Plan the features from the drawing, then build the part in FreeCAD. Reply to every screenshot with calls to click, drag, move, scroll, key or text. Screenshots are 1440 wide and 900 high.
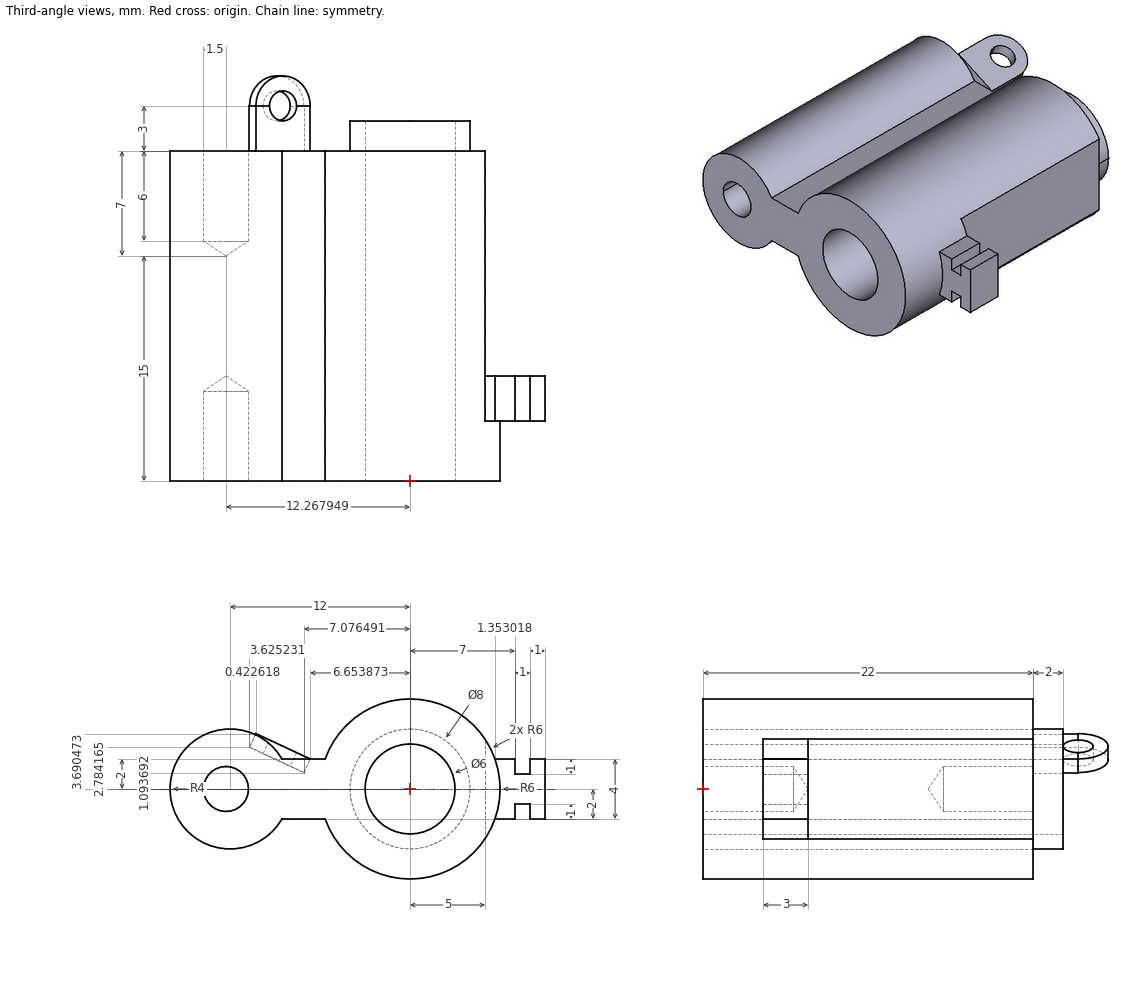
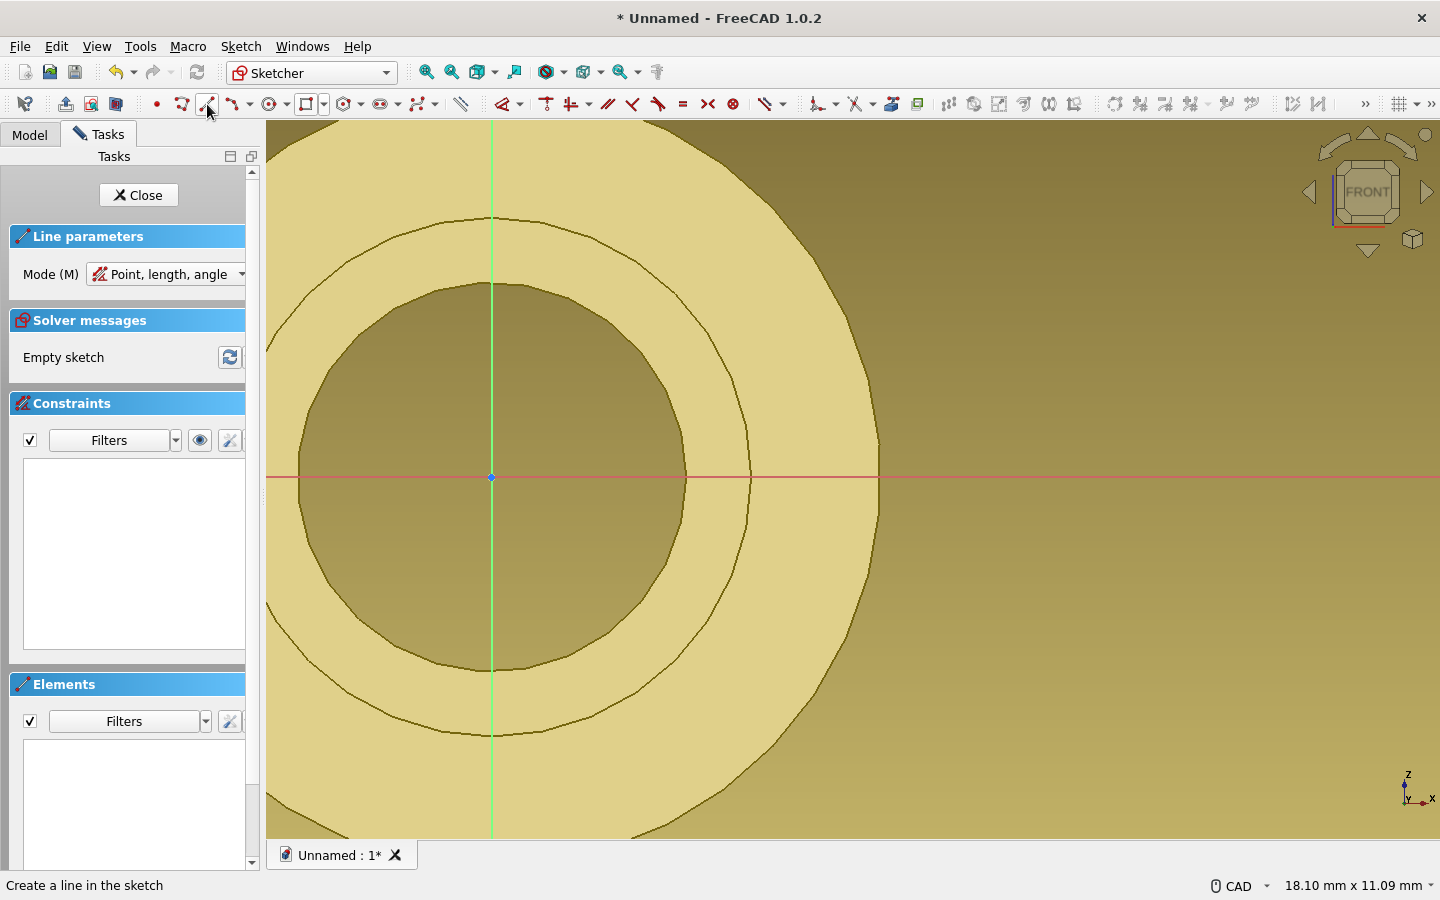
click(816, 692)
click(816, 262)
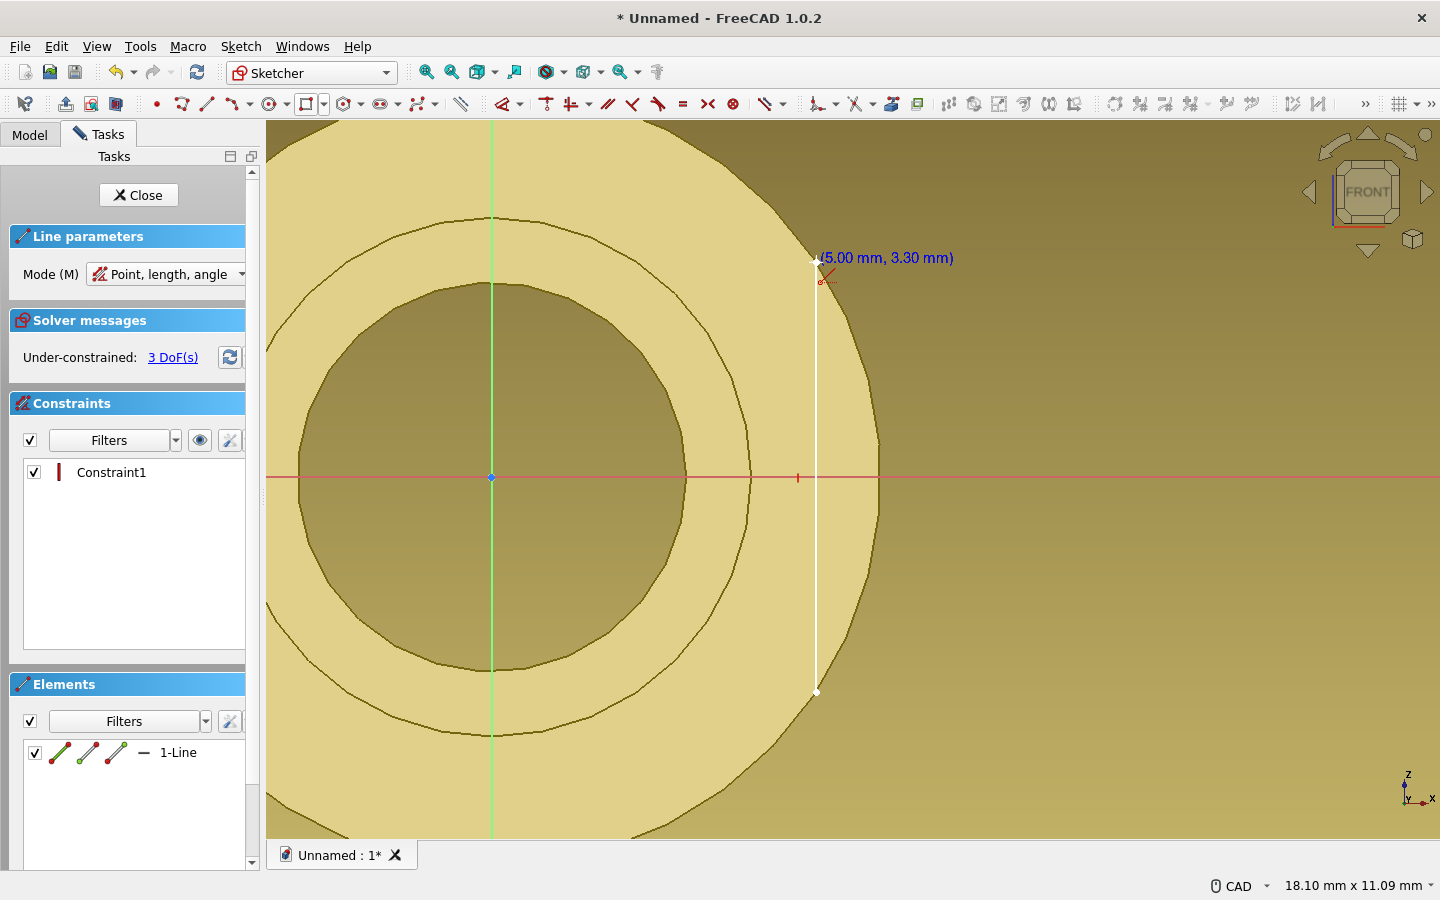
click(182, 104)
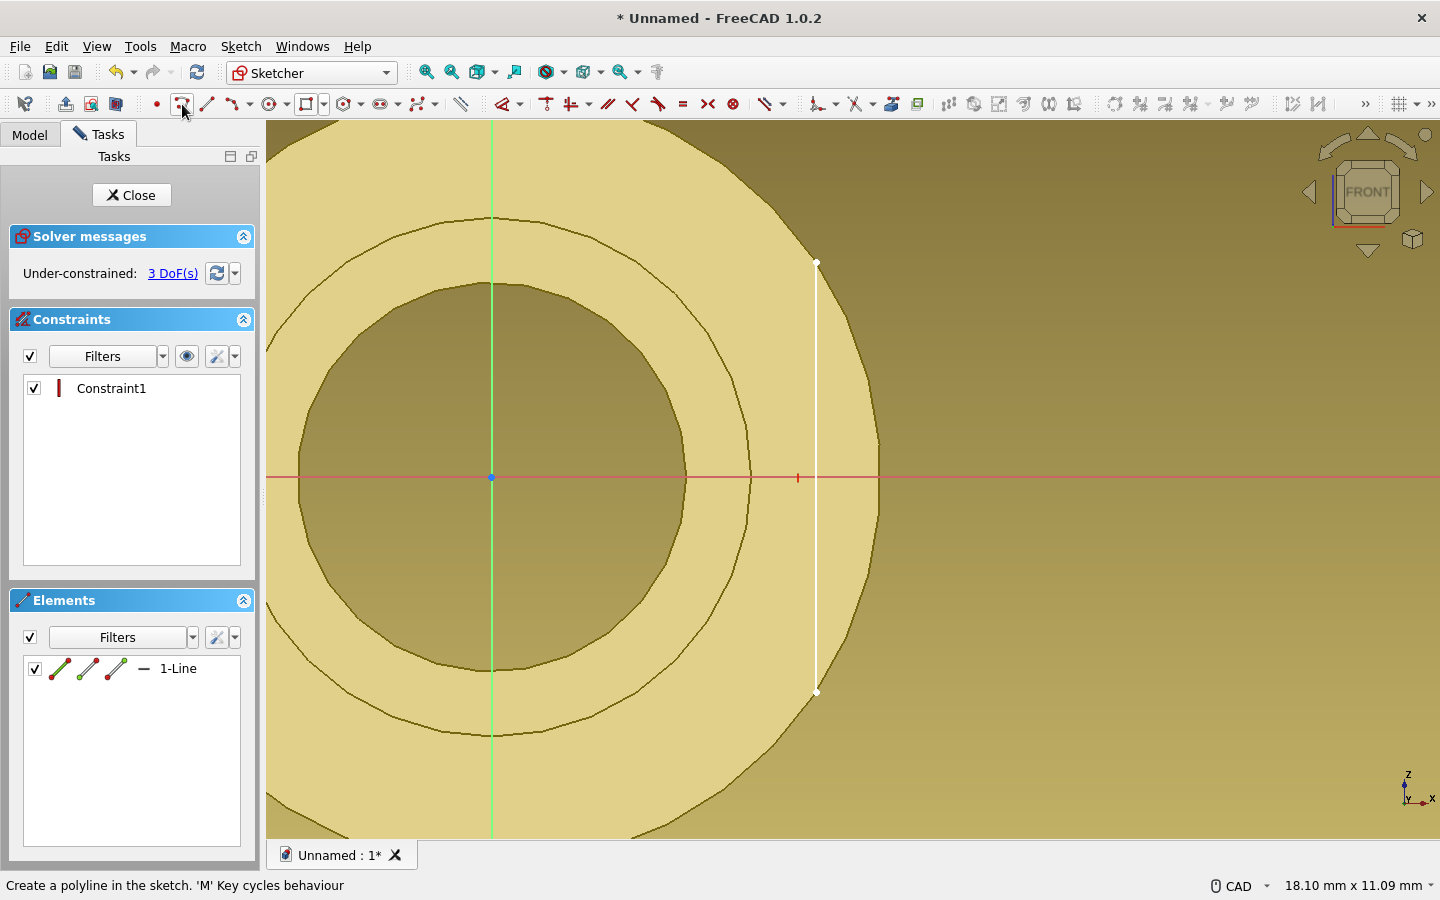
click(858, 346)
click(946, 346)
click(946, 412)
click(1011, 412)
click(1011, 347)
click(1075, 347)
click(1075, 607)
click(1011, 607)
click(1011, 542)
click(946, 542)
click(946, 607)
click(859, 607)
right_click(859, 607)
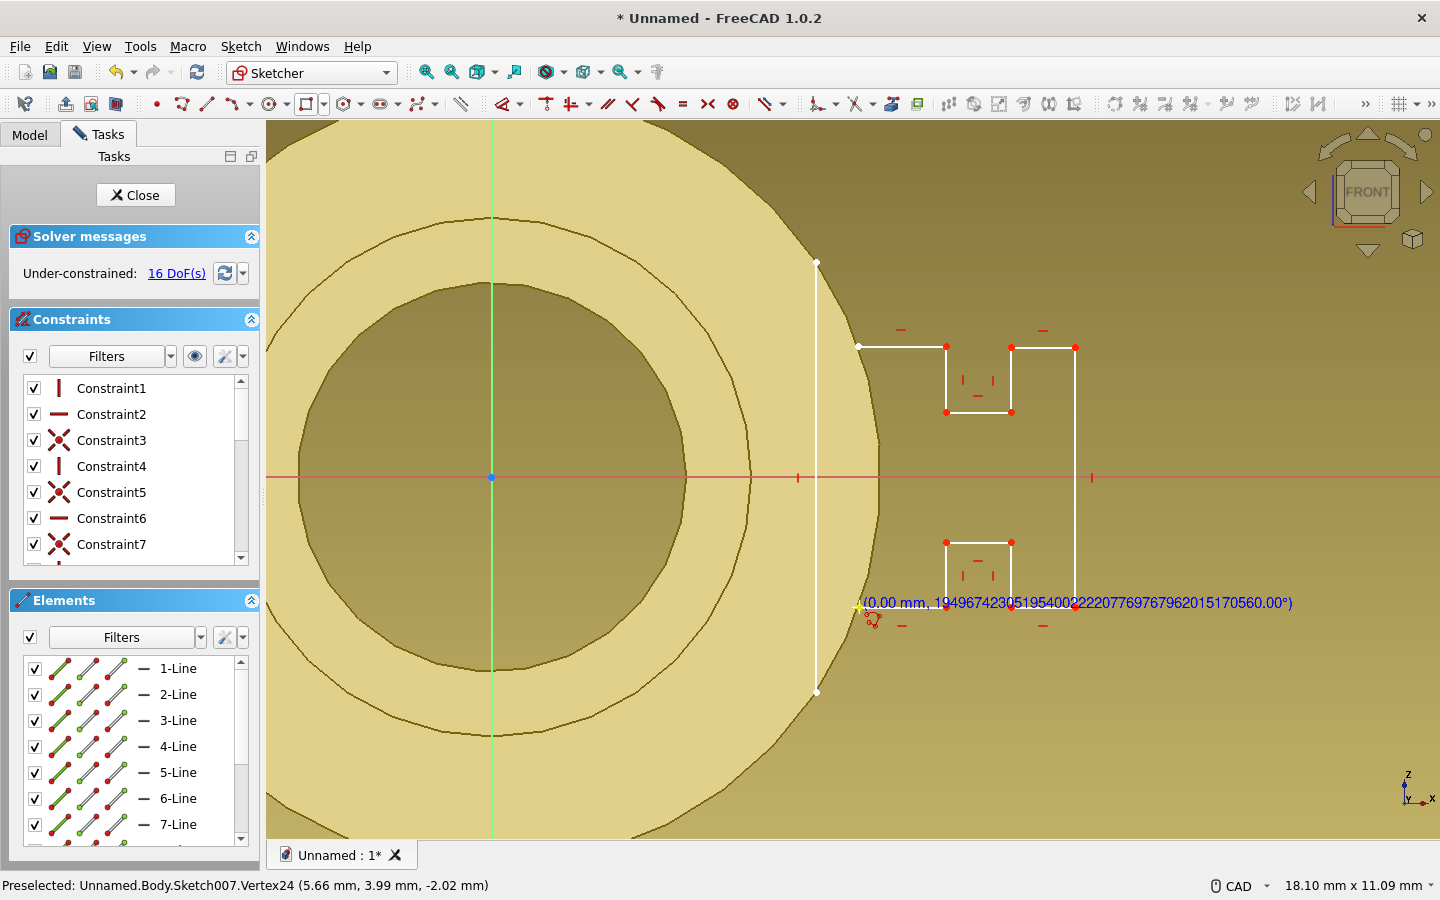
click(232, 104)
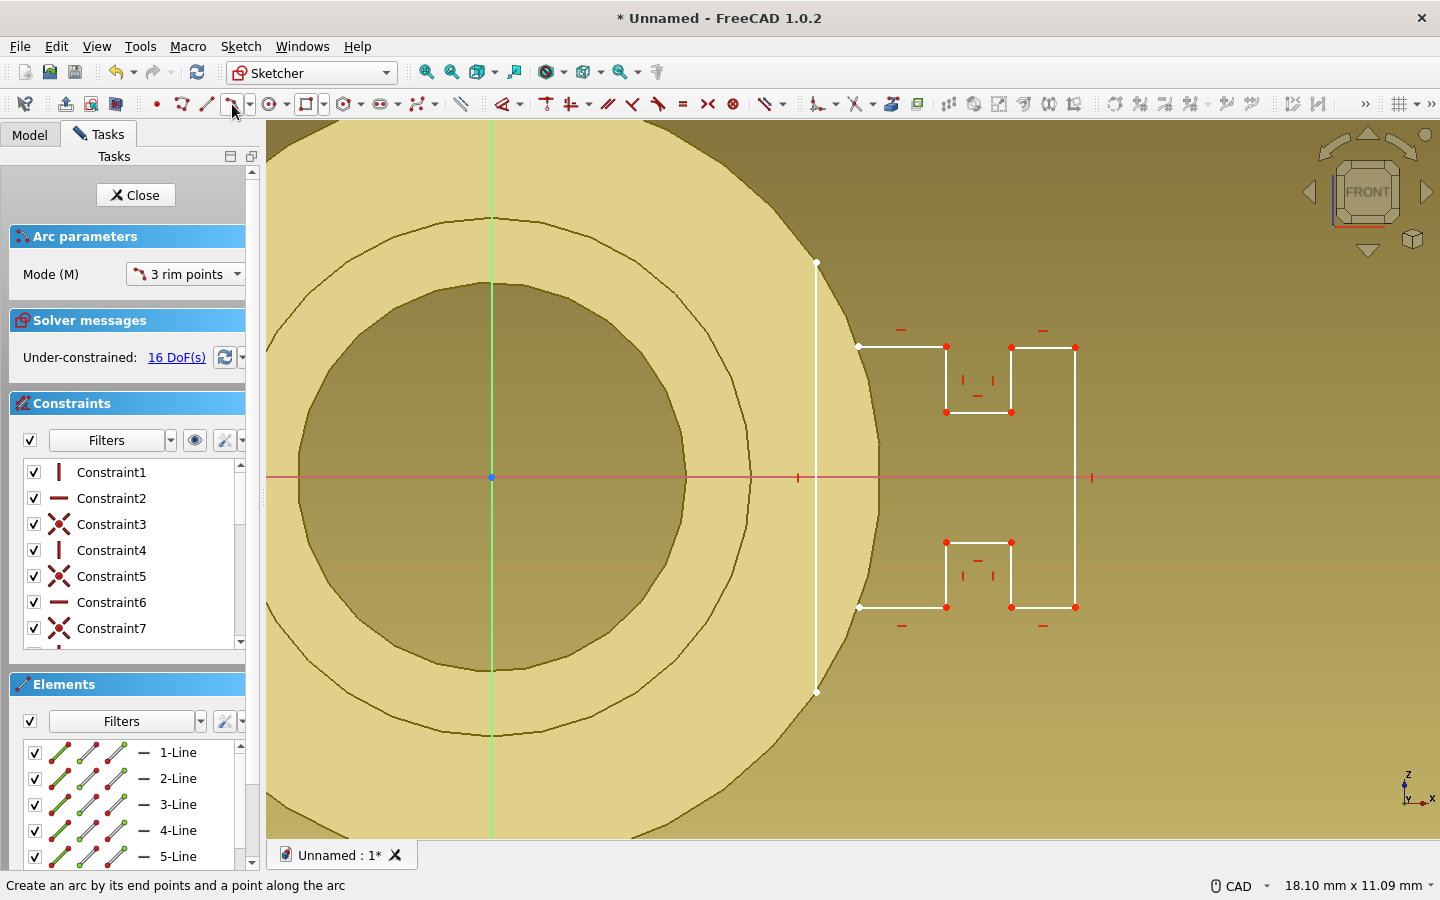
click(816, 263)
click(858, 347)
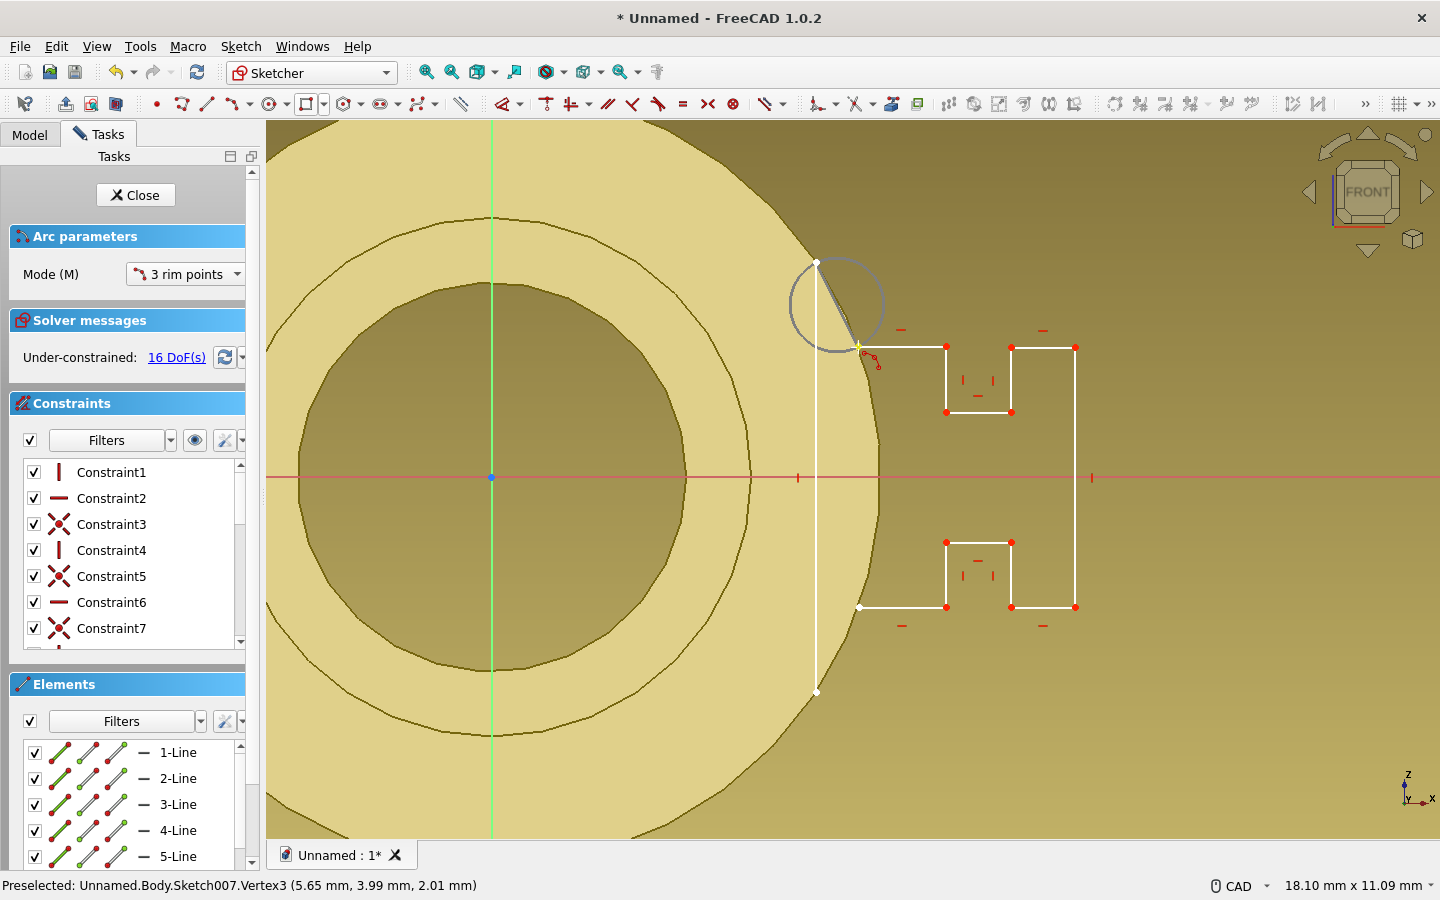
scroll(840, 303, up, 9)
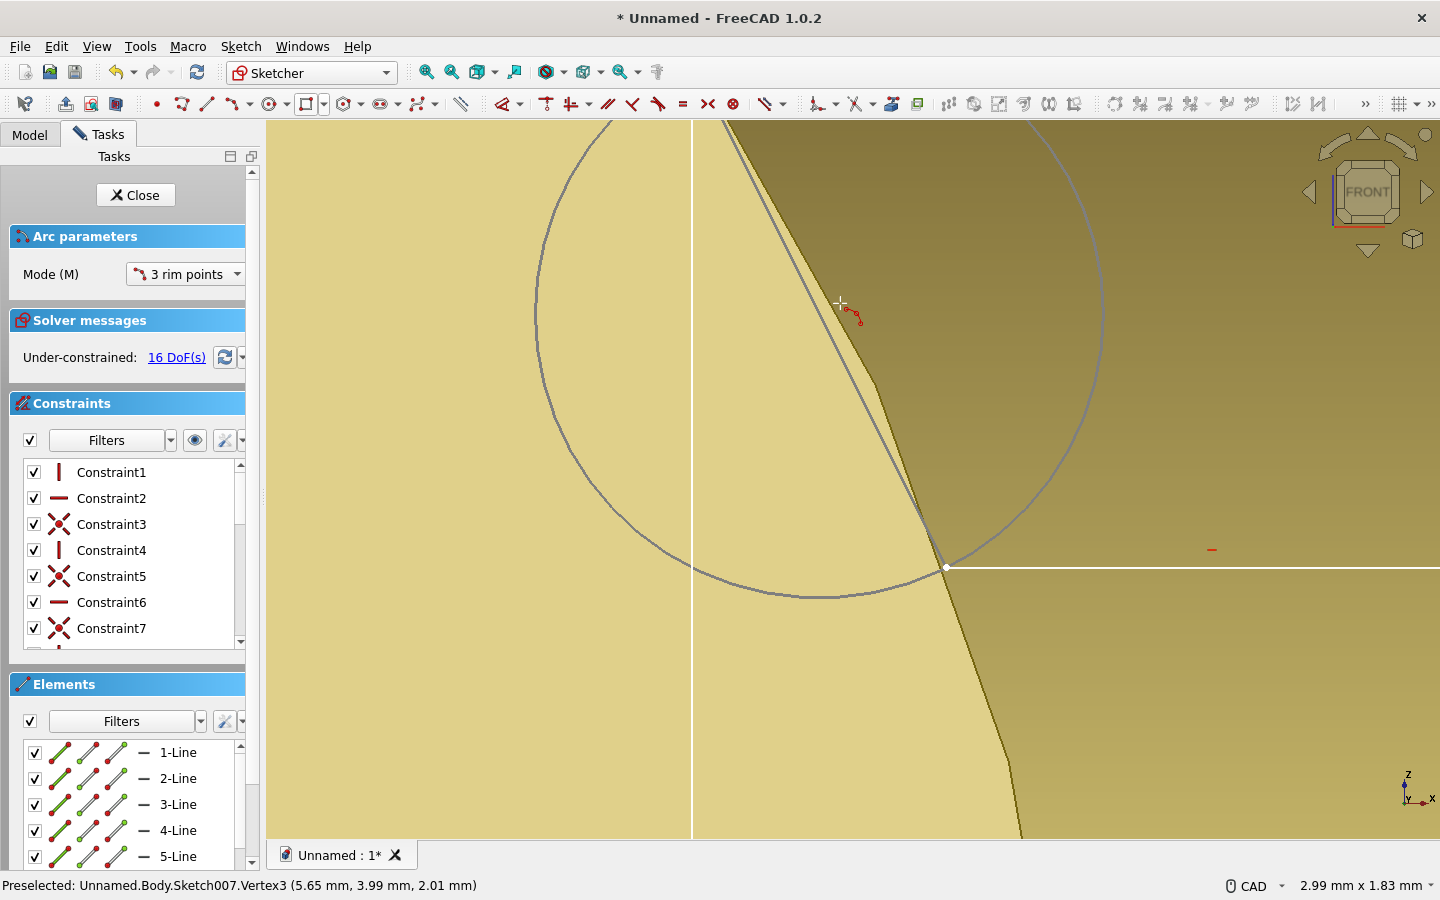
click(835, 299)